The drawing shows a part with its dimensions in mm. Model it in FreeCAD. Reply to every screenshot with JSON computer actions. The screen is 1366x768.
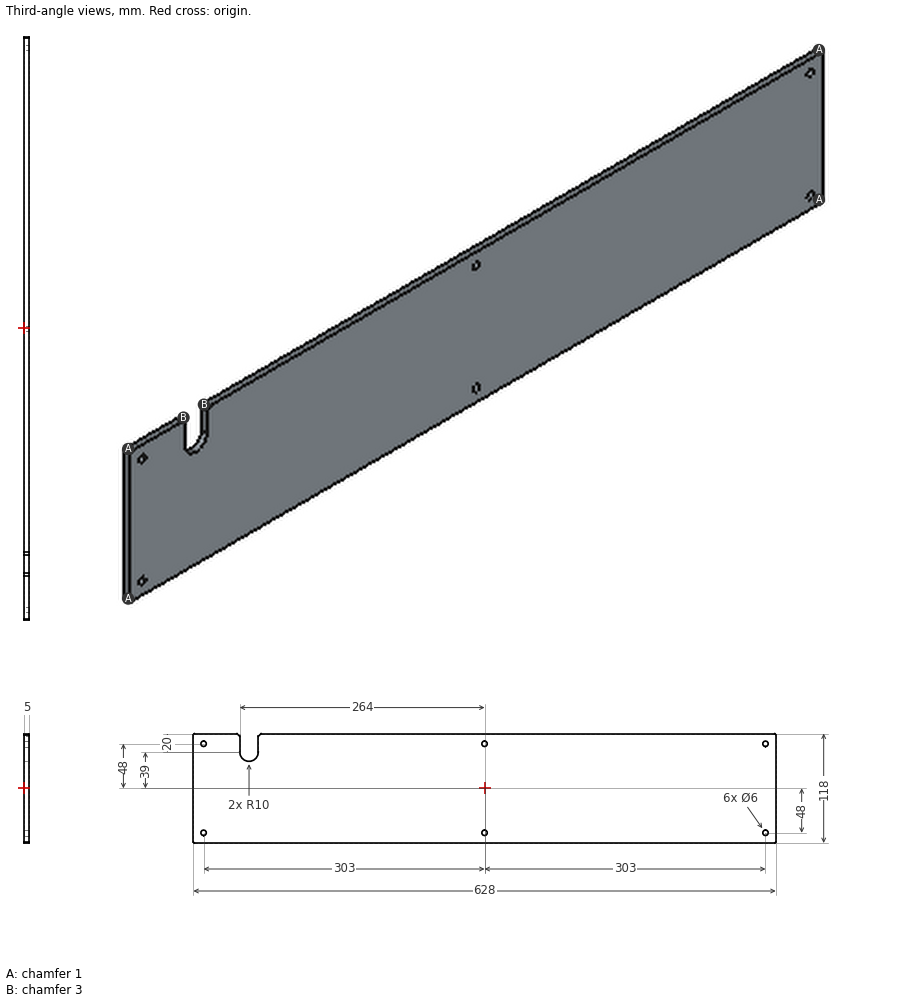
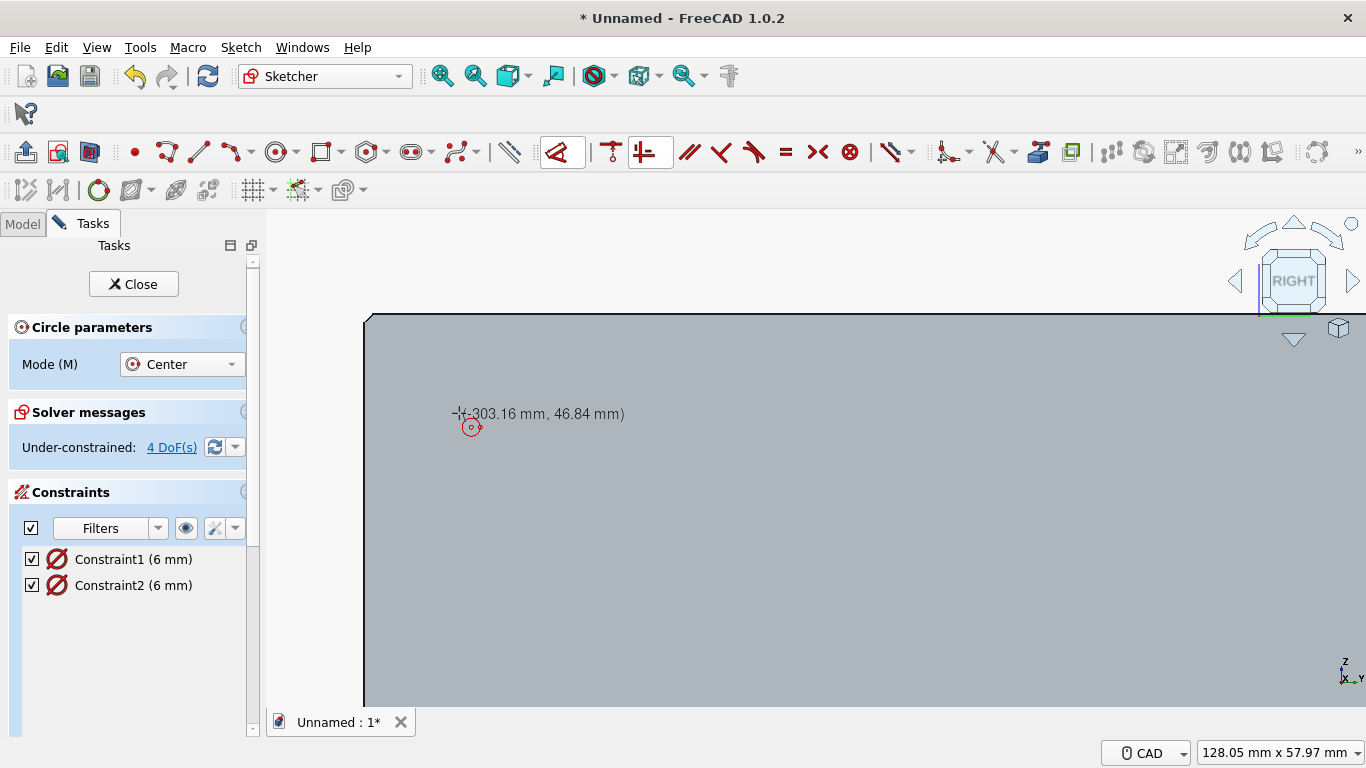
{"action": "scroll", "coordinate": [459, 413], "scroll_direction": "down", "scroll_amount": 11}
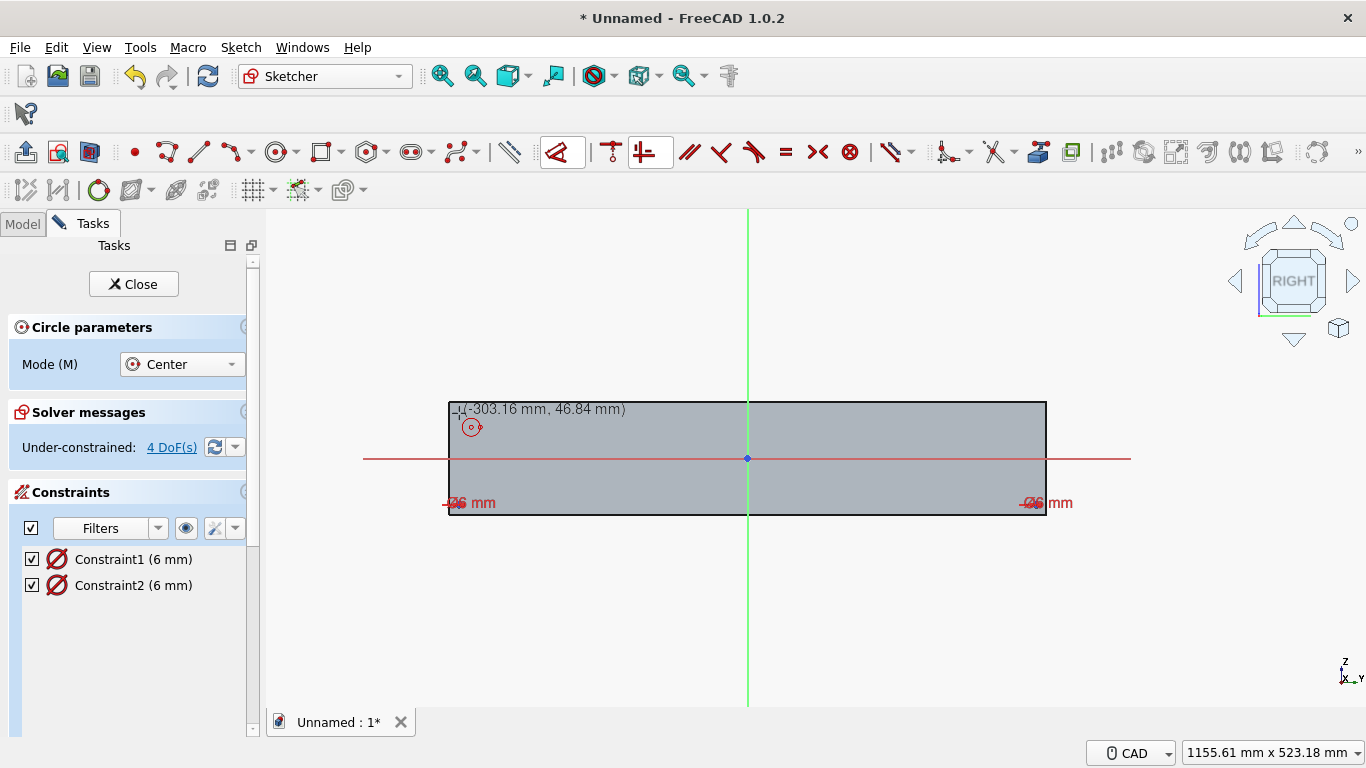
{"action": "left_click", "coordinate": [459, 413]}
{"action": "mouse_move", "coordinate": [461, 411]}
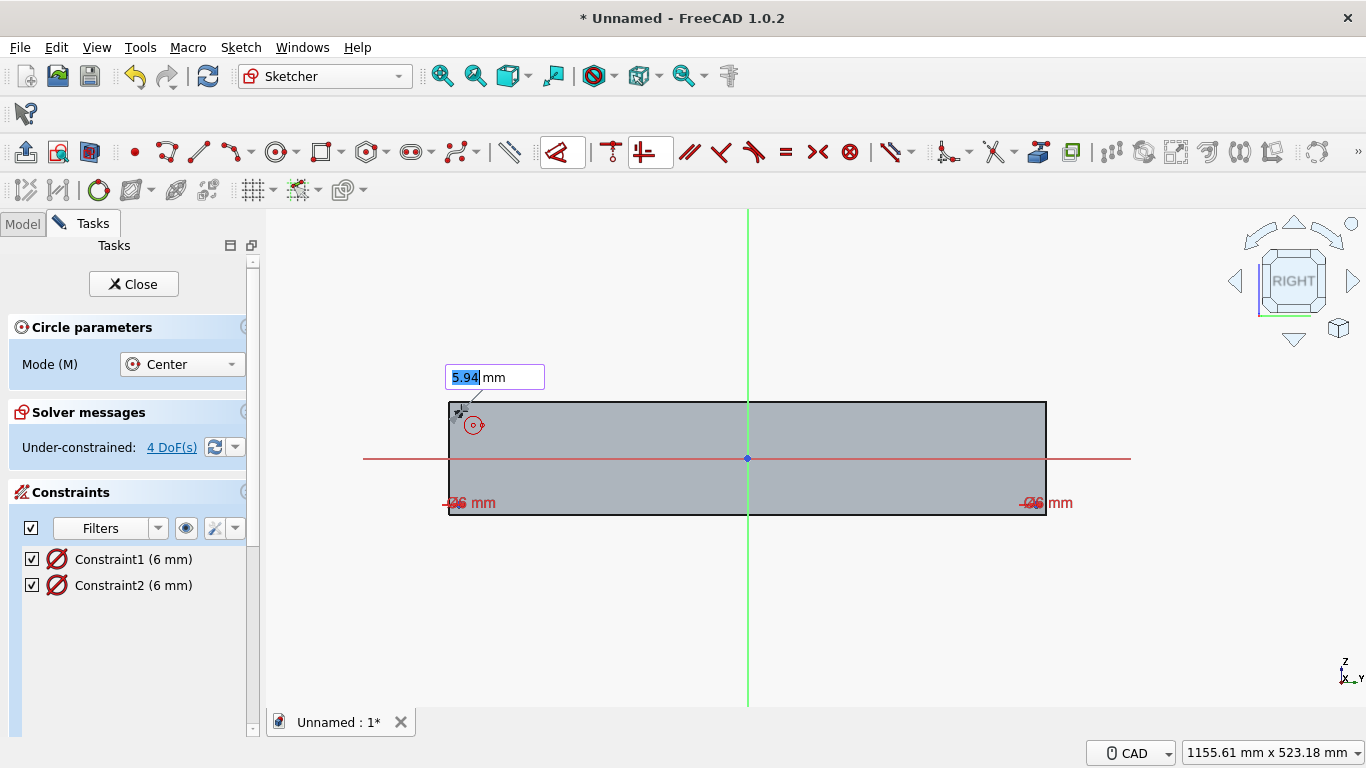
{"action": "type", "text": "6"}
{"action": "key", "text": "Return"}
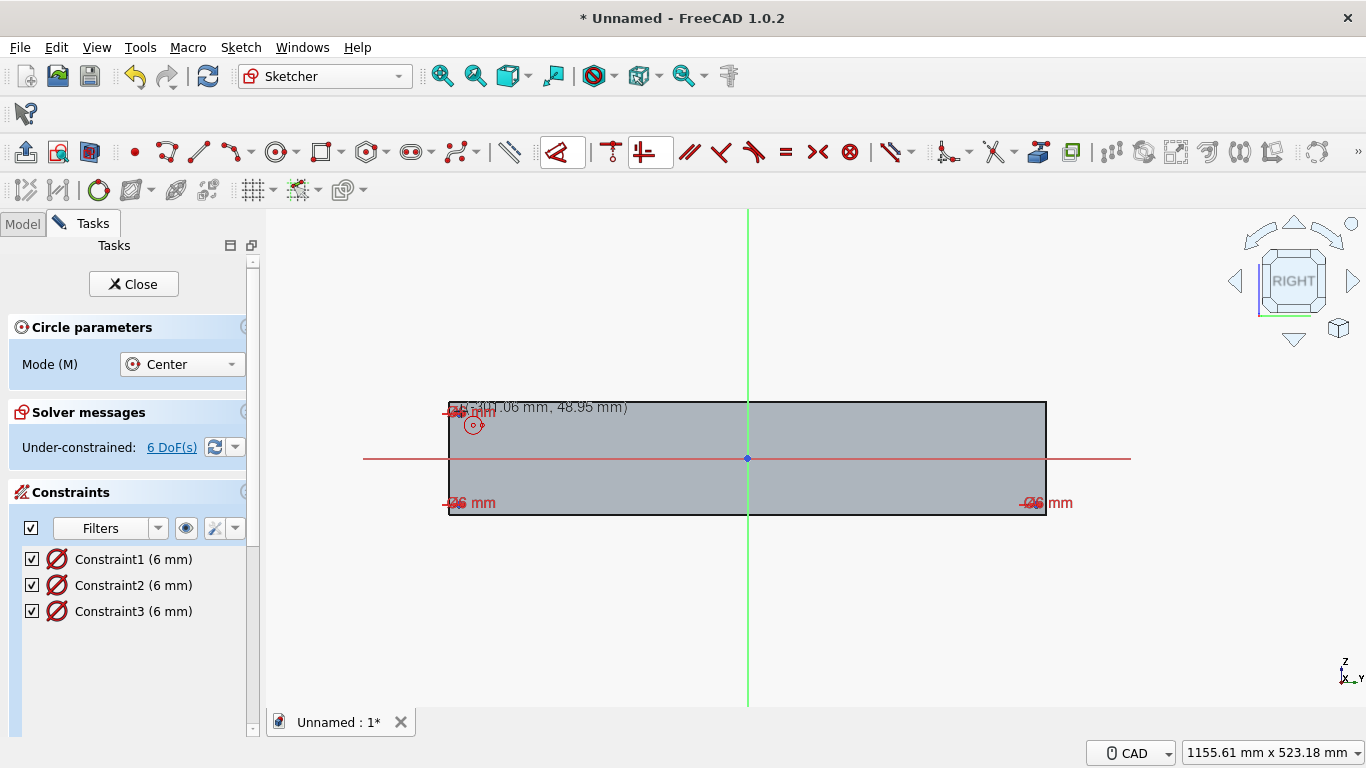
{"action": "scroll", "coordinate": [1036, 413], "scroll_direction": "up", "scroll_amount": 11}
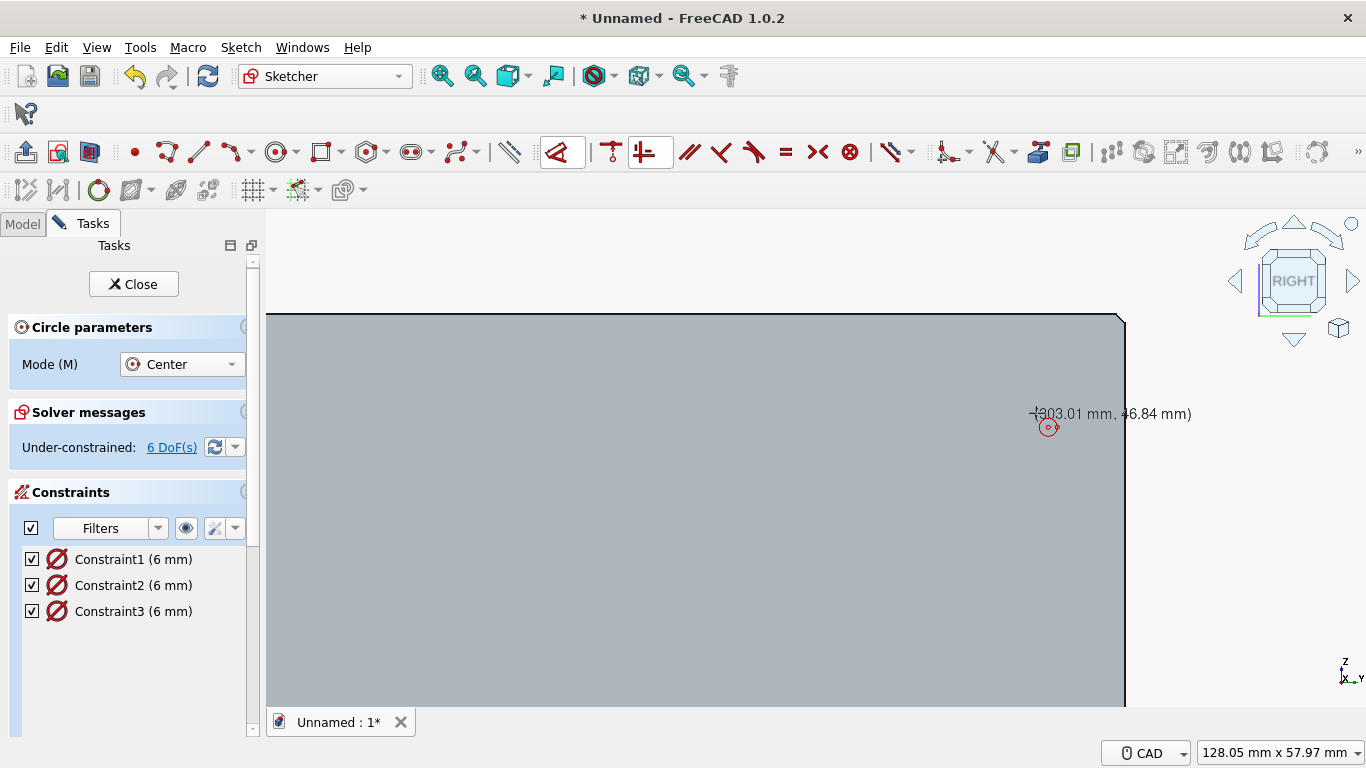
{"action": "scroll", "coordinate": [1037, 413], "scroll_direction": "down", "scroll_amount": 11}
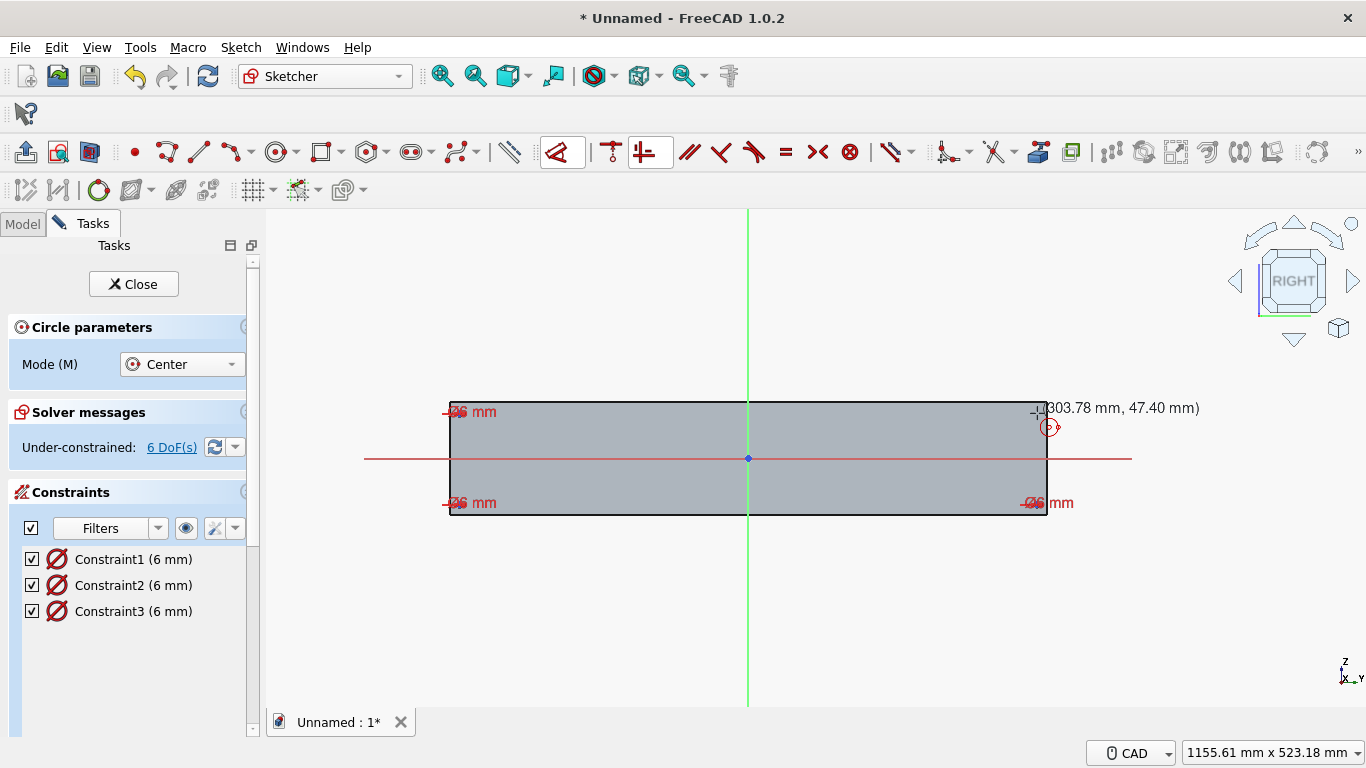
{"action": "left_click", "coordinate": [1037, 413]}
{"action": "mouse_move", "coordinate": [1039, 411]}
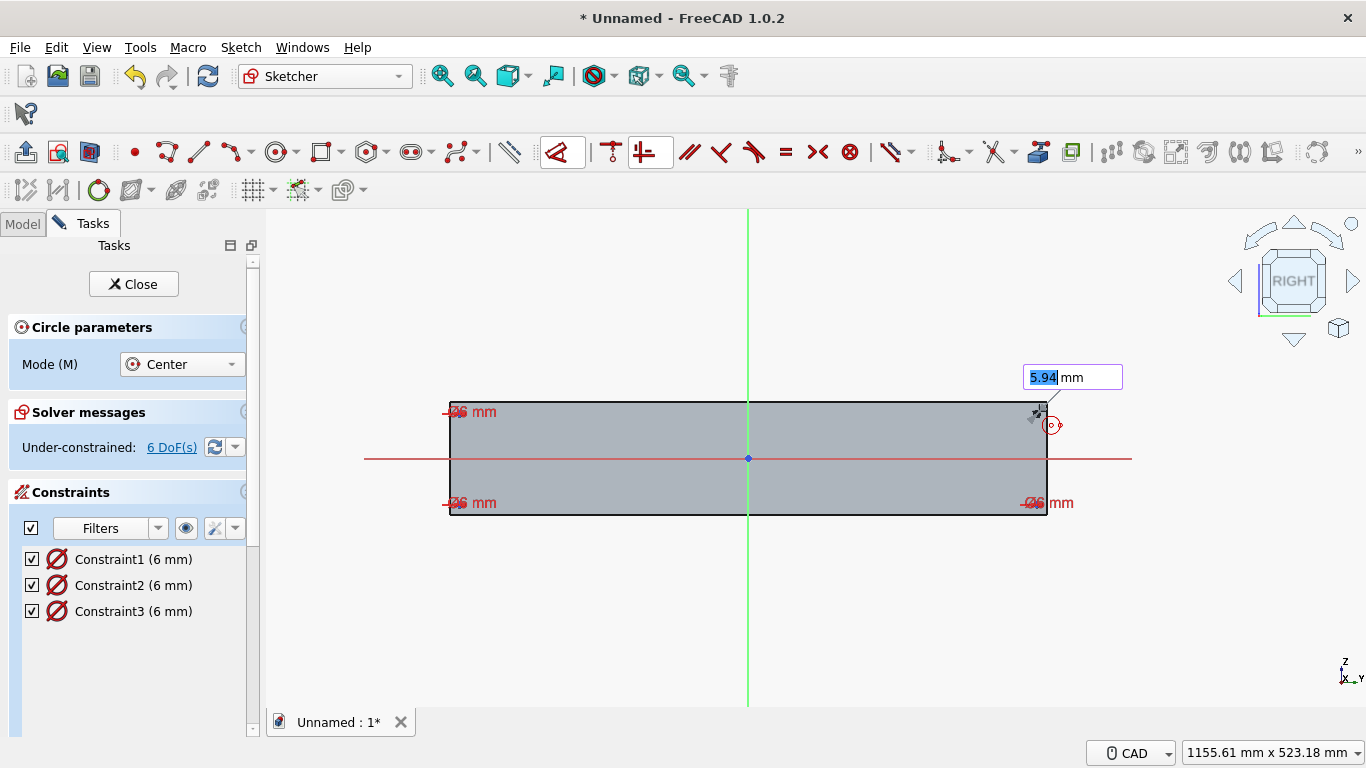
{"action": "type", "text": "6"}
{"action": "key", "text": "Return"}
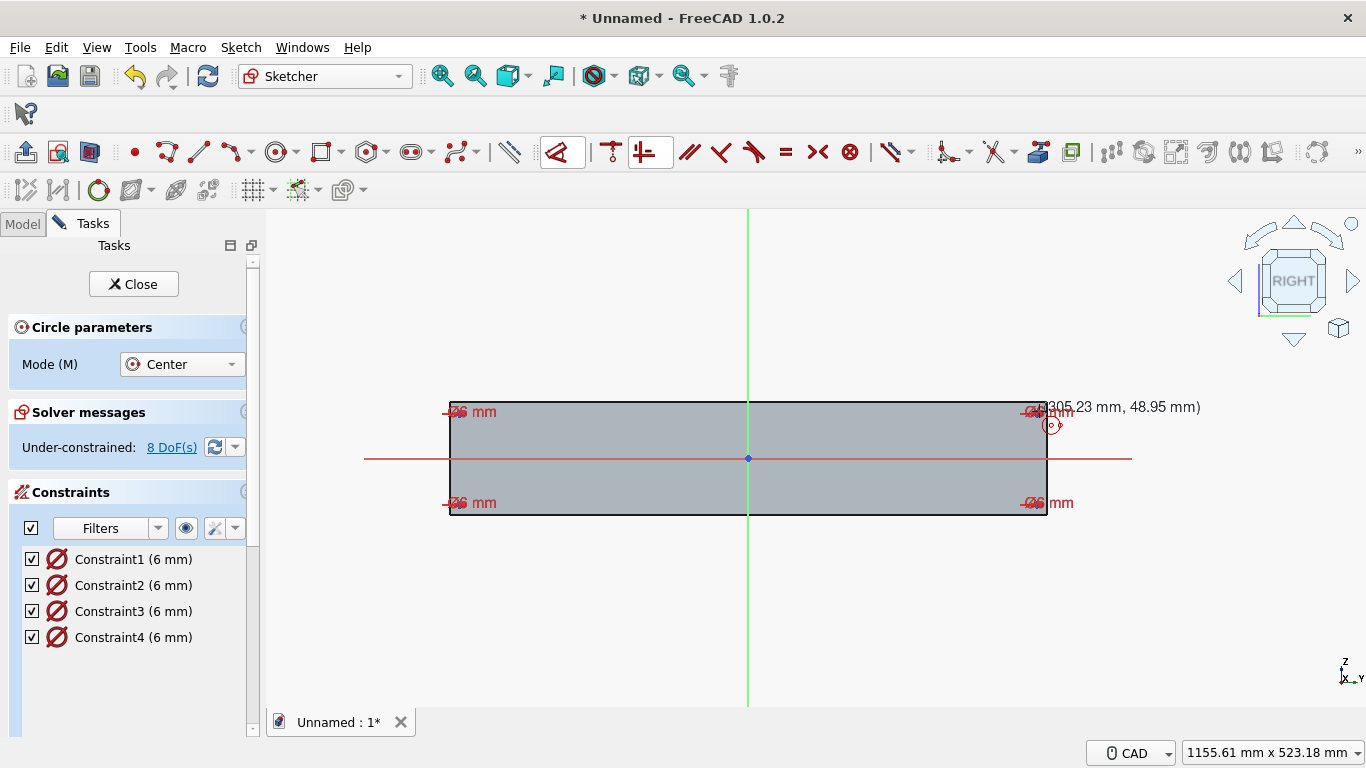
{"action": "scroll", "coordinate": [748, 413], "scroll_direction": "up", "scroll_amount": 11}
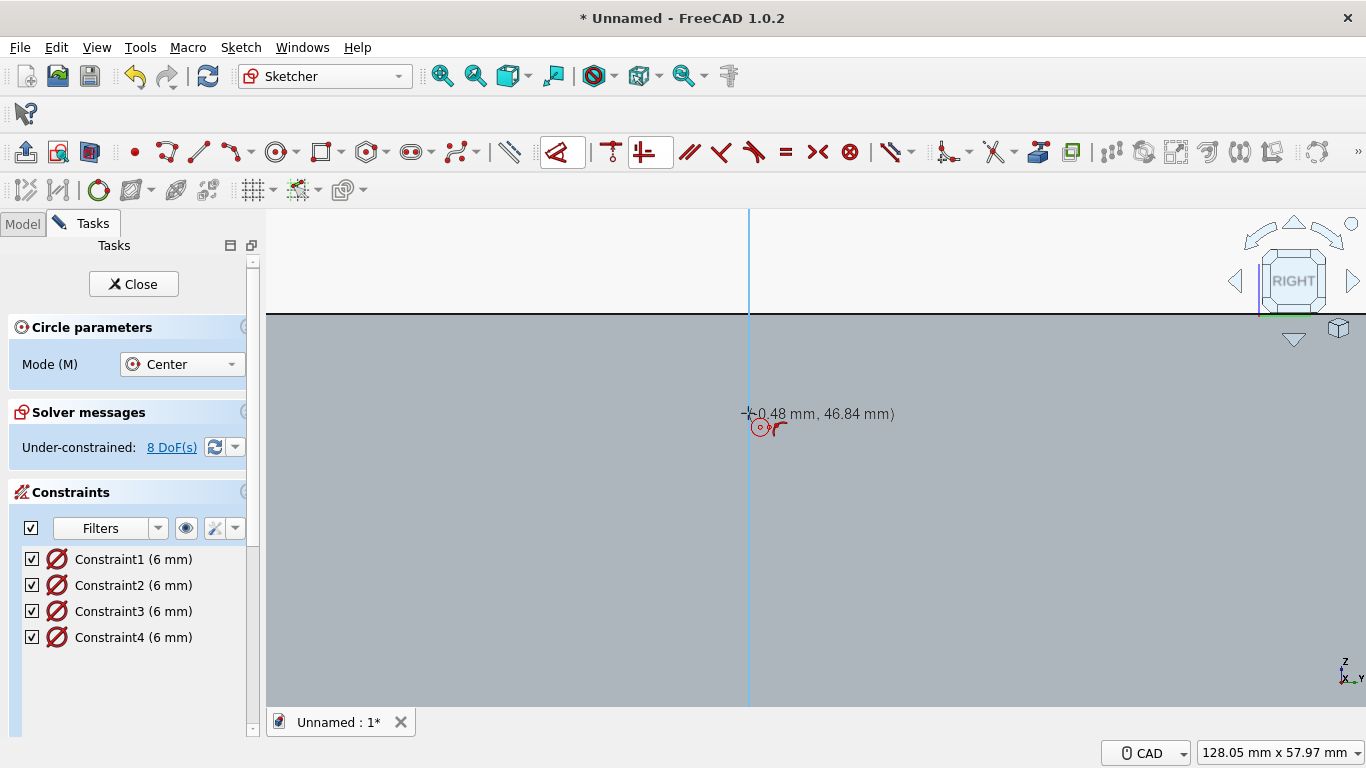
{"action": "scroll", "coordinate": [747, 413], "scroll_direction": "down", "scroll_amount": 11}